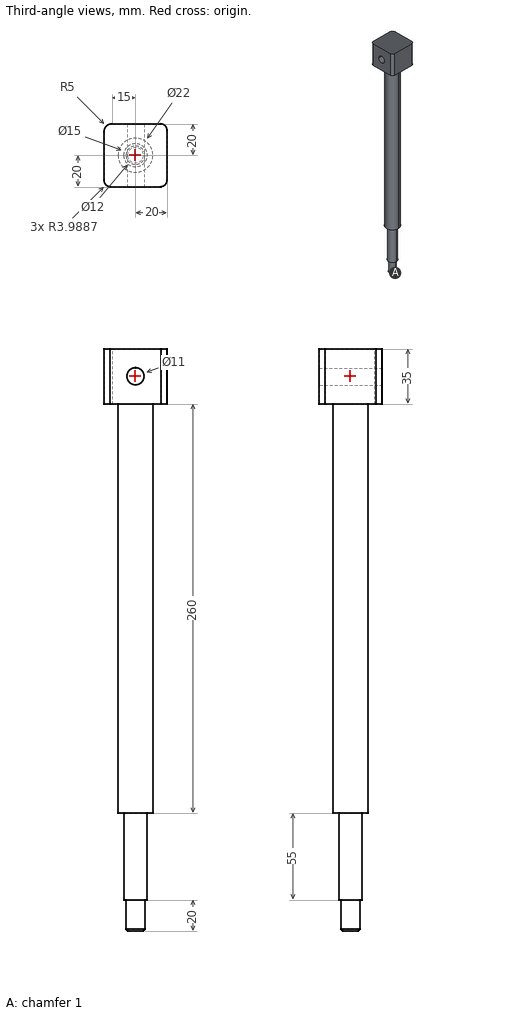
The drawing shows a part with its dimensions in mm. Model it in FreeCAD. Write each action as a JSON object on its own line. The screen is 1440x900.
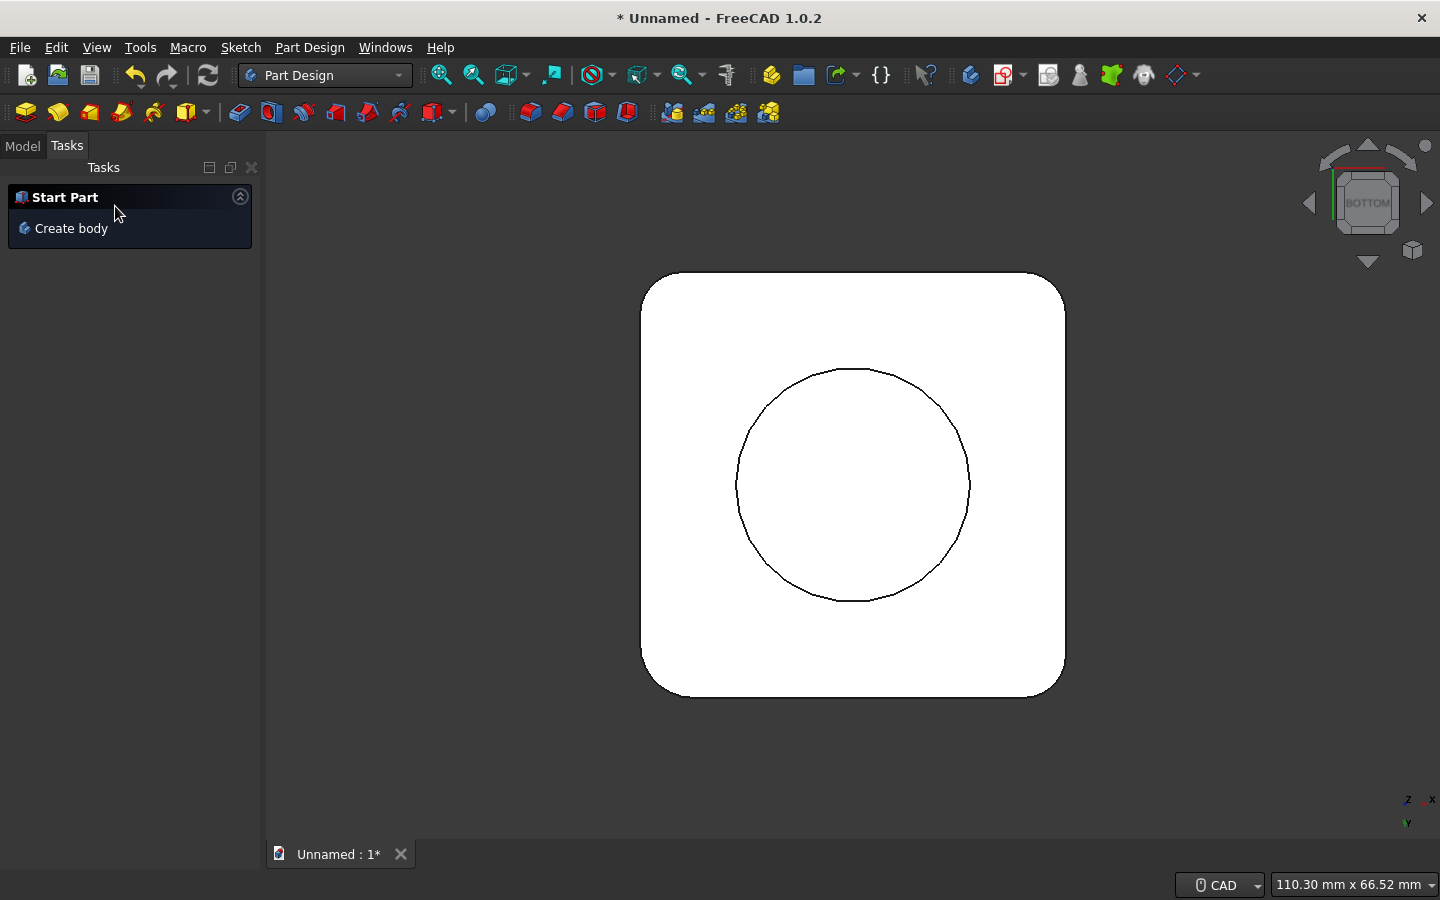
{"action": "left_click", "coordinate": [853, 484]}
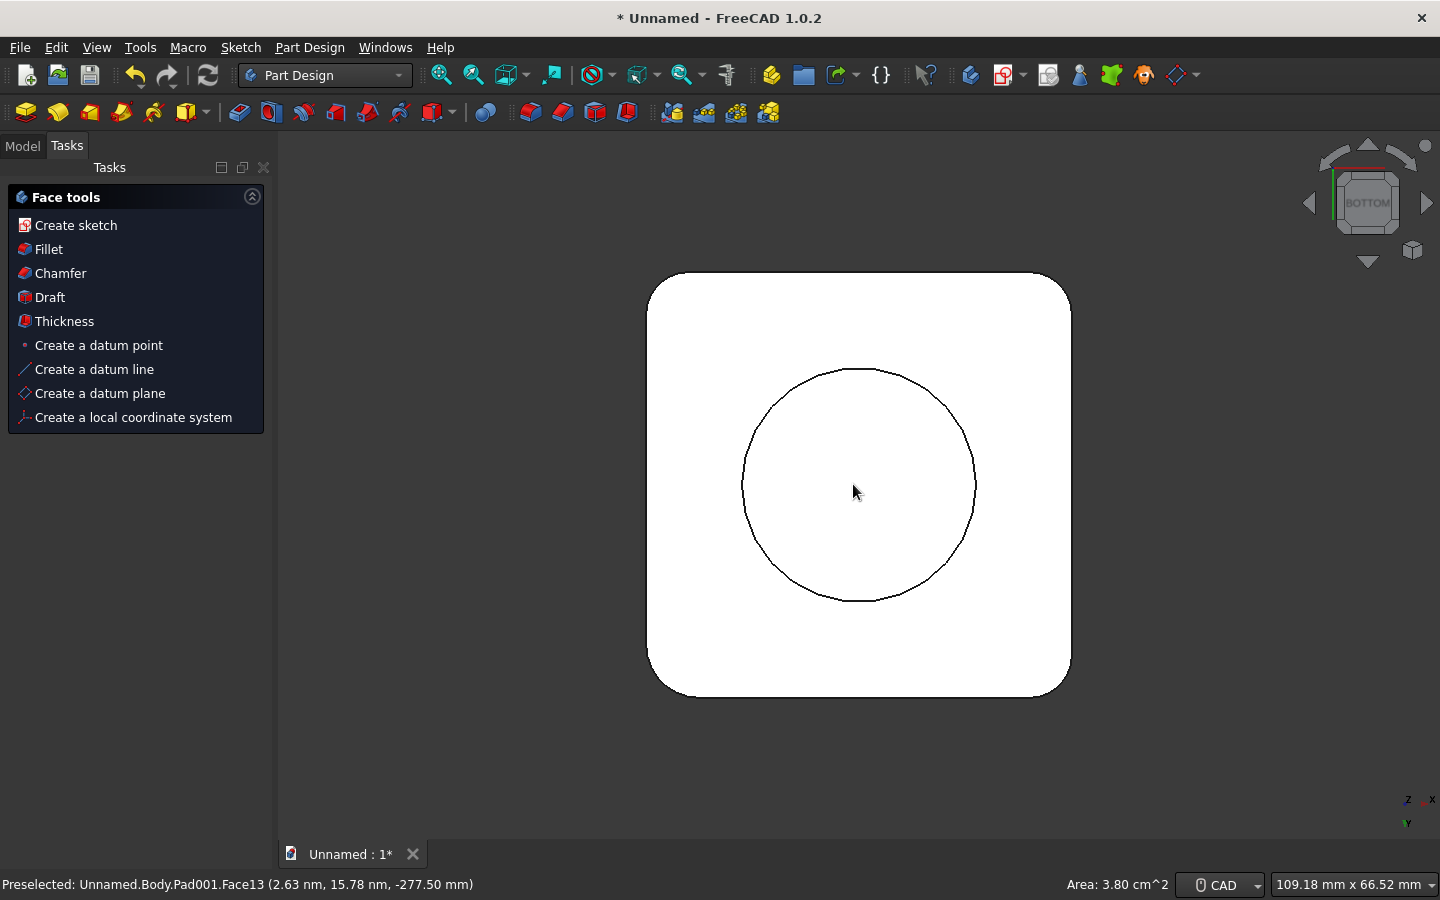
{"action": "left_click", "coordinate": [1004, 76]}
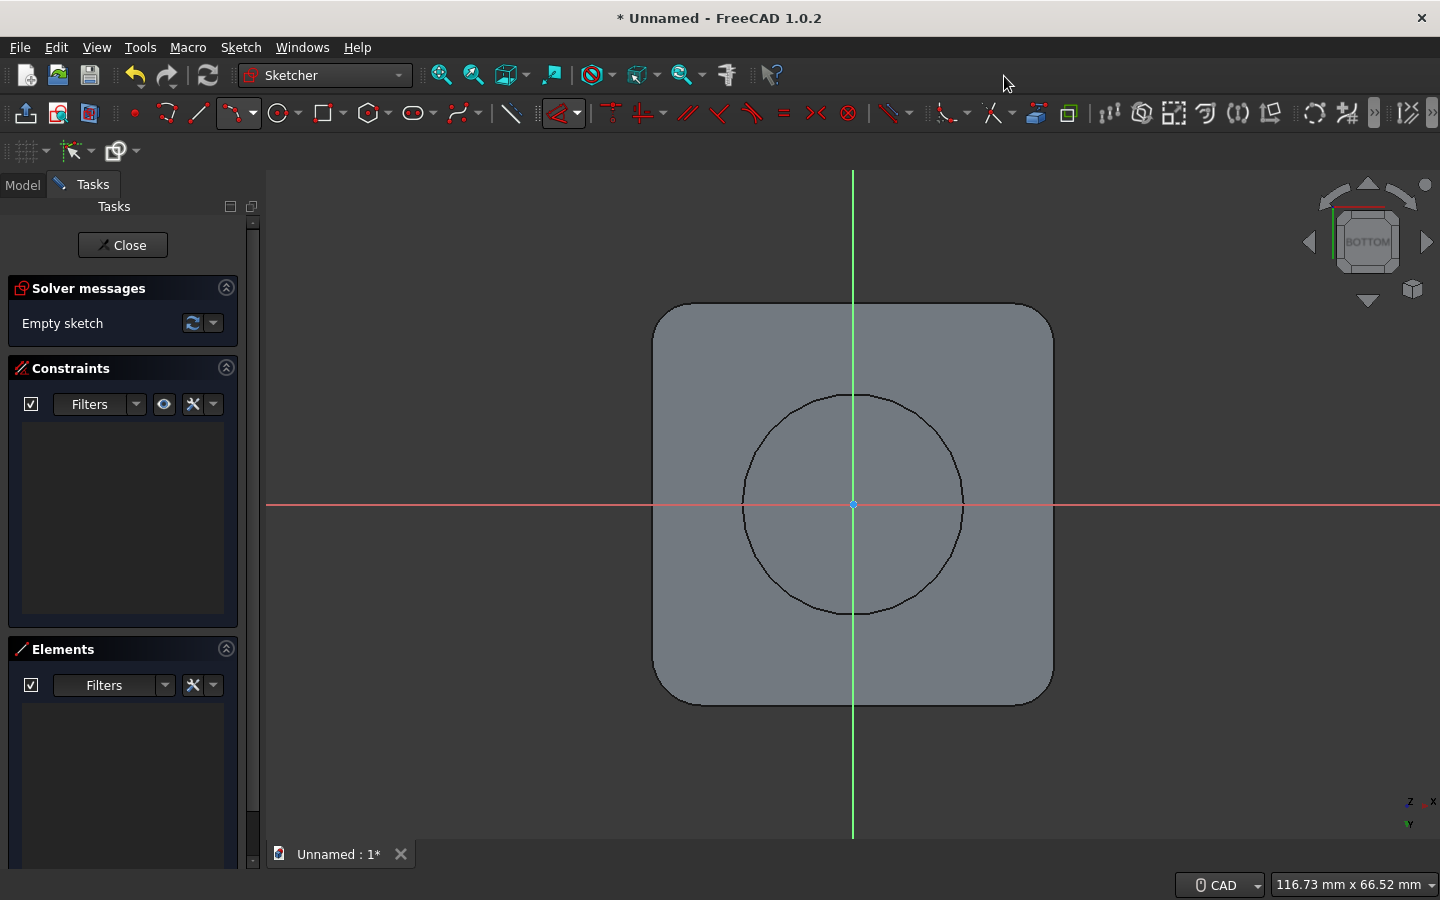
{"action": "scroll", "coordinate": [893, 505], "scroll_direction": "up", "scroll_amount": 5}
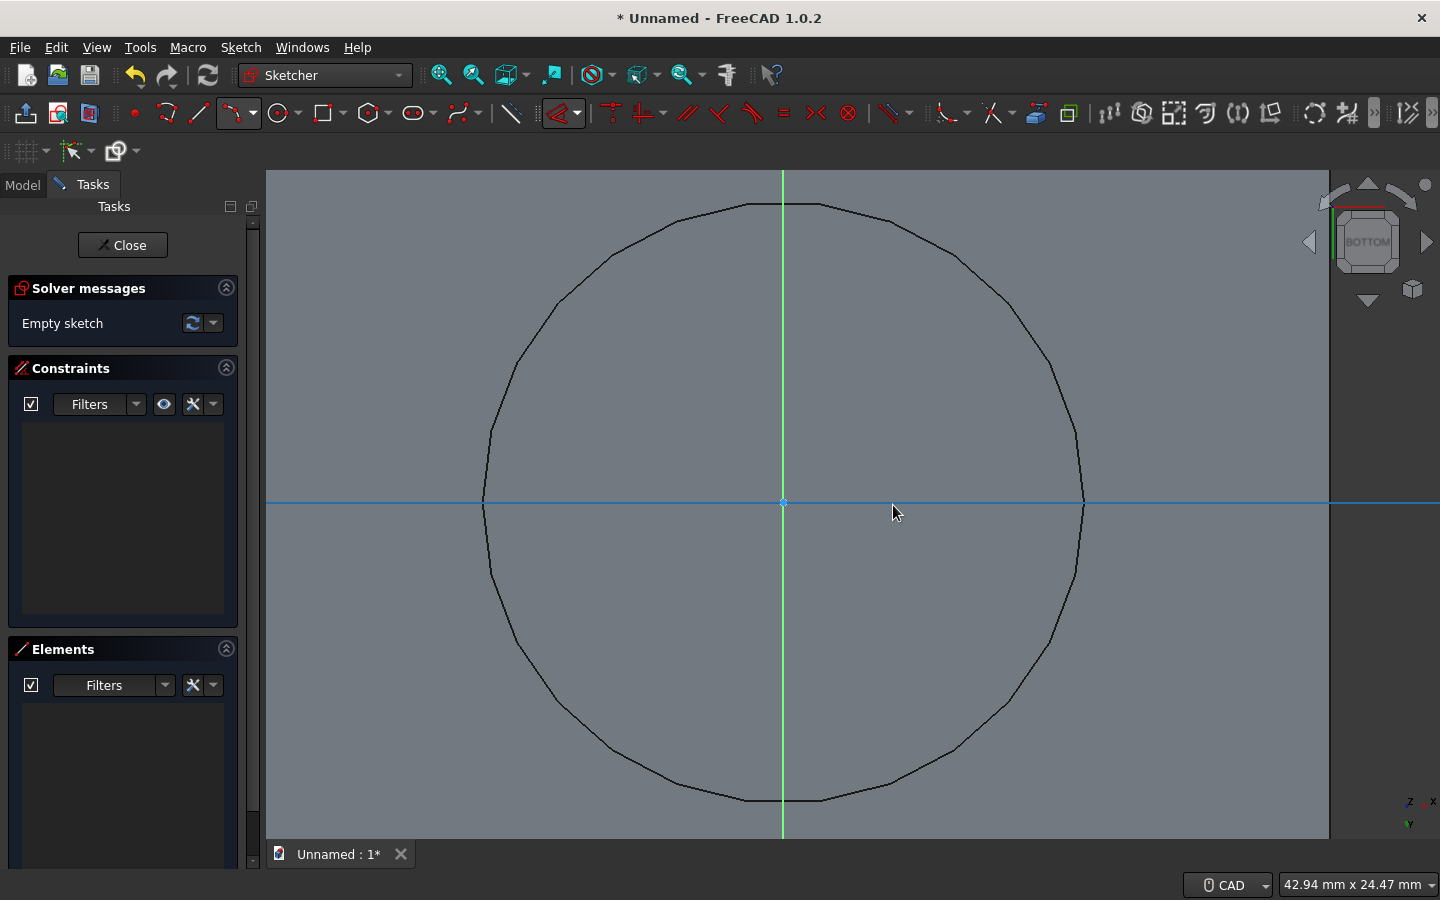
{"action": "left_click", "coordinate": [278, 114]}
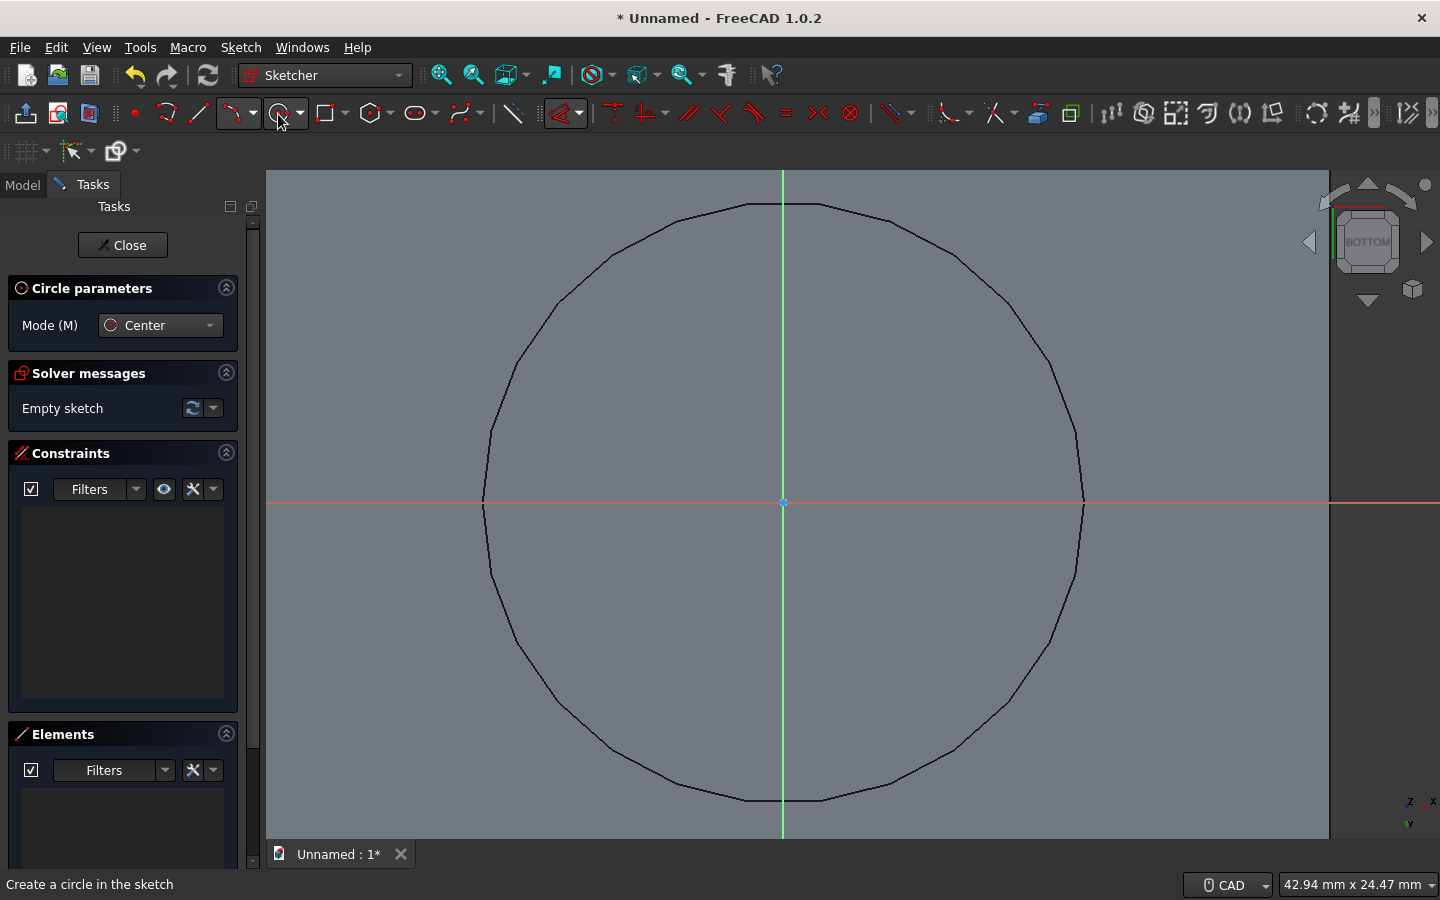
{"action": "left_click", "coordinate": [783, 503]}
{"action": "left_click", "coordinate": [928, 358]}
{"action": "key", "text": "Escape"}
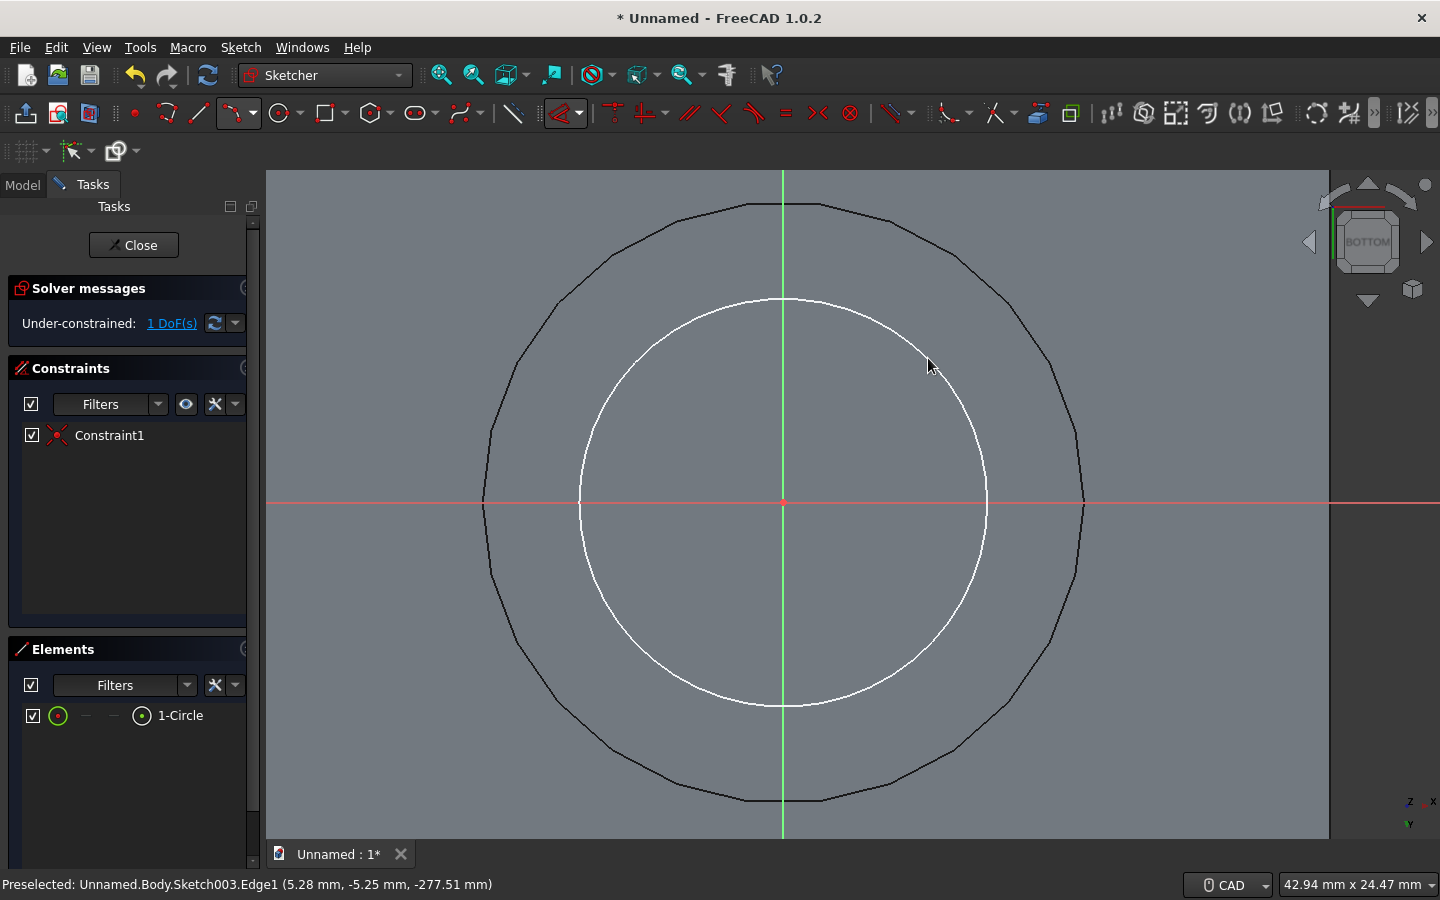
{"action": "left_click", "coordinate": [927, 358]}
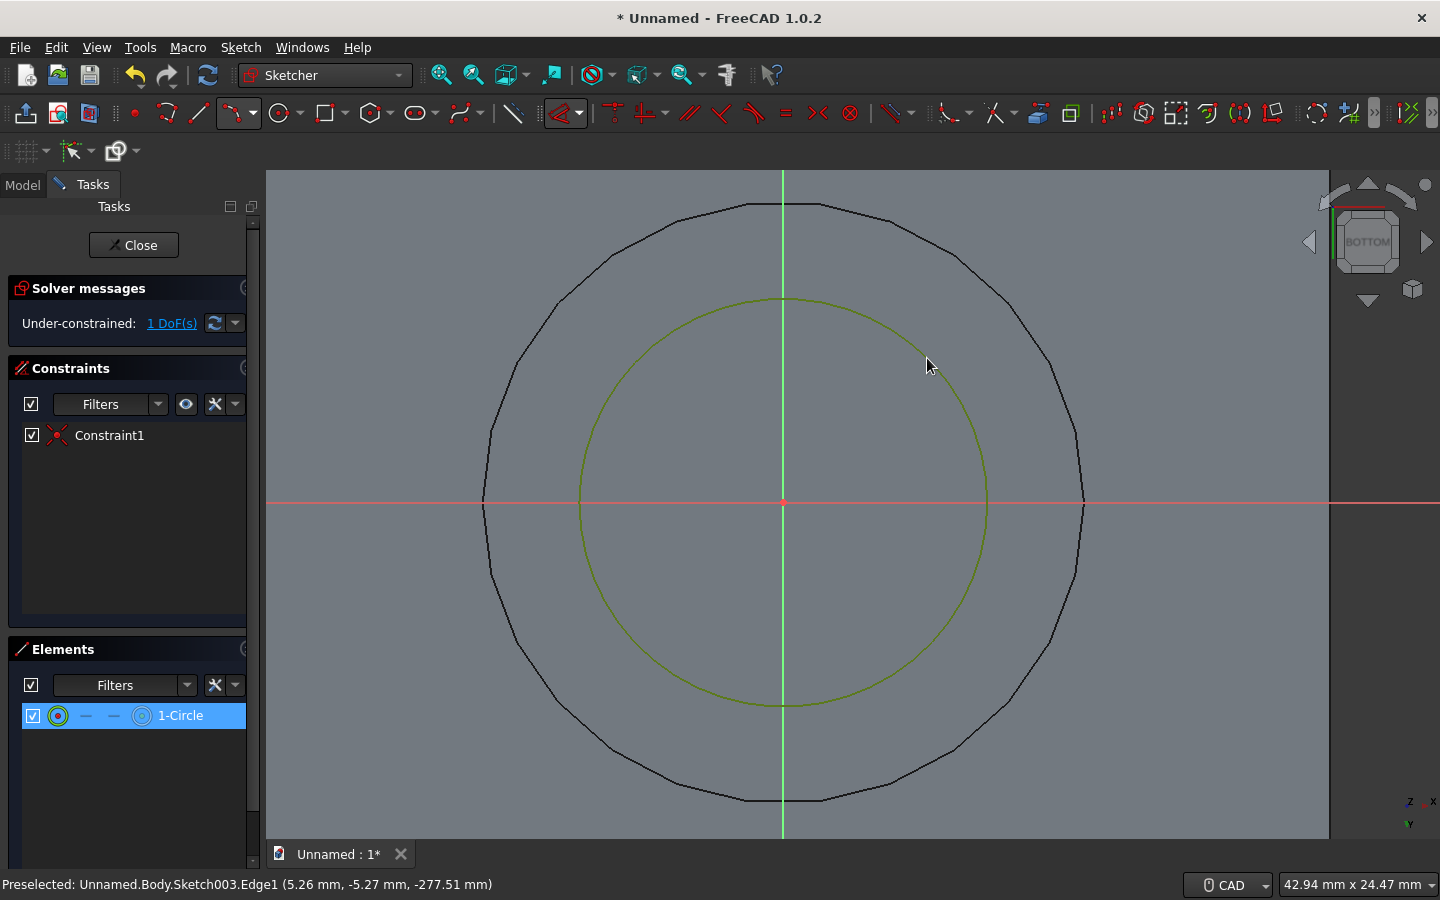
{"action": "left_click", "coordinate": [582, 114]}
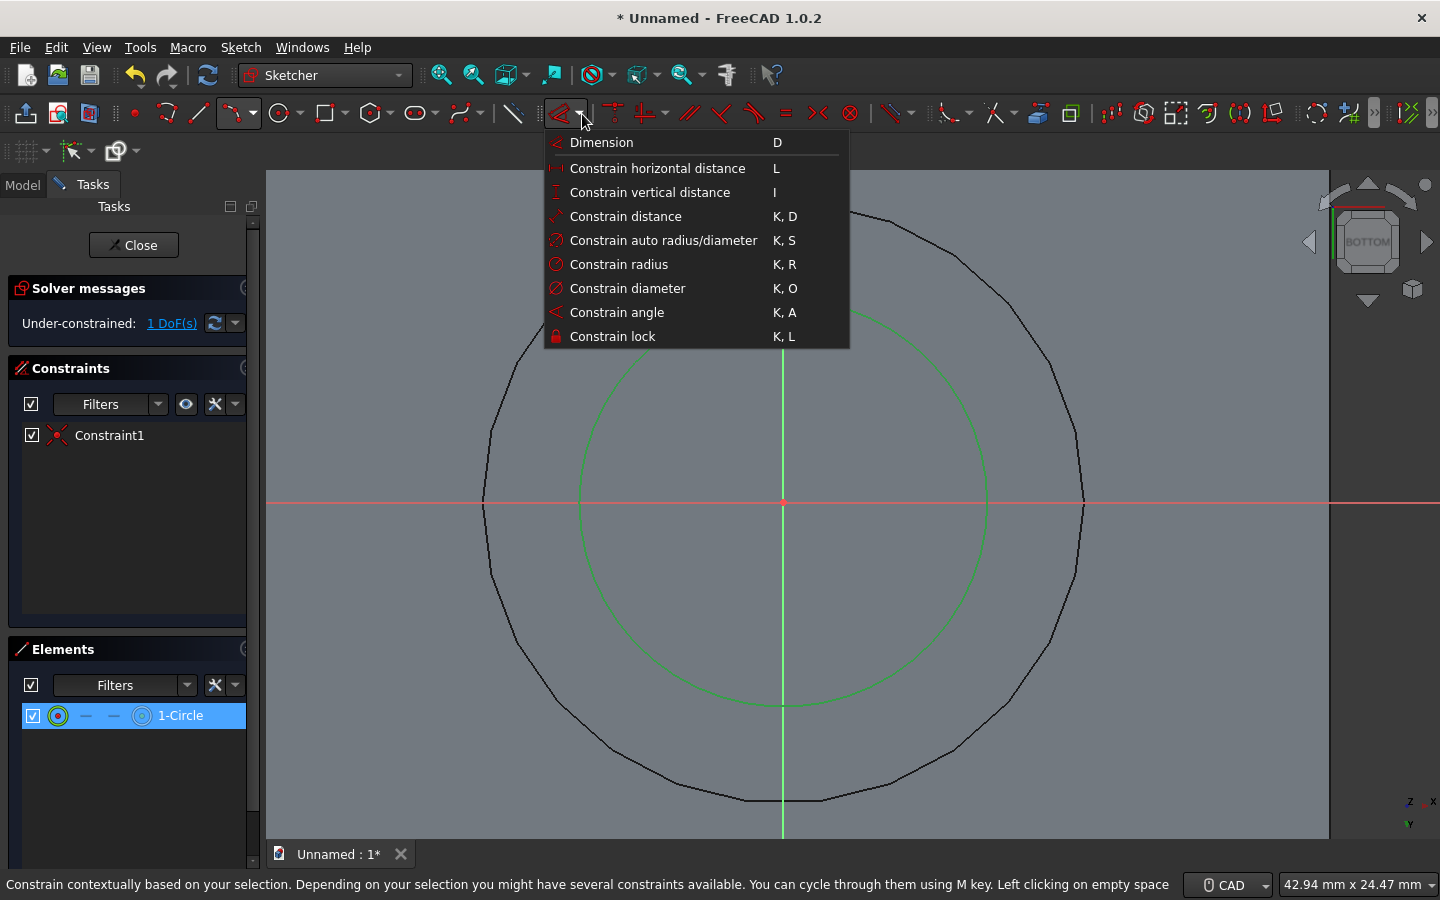
{"action": "left_click", "coordinate": [697, 288]}